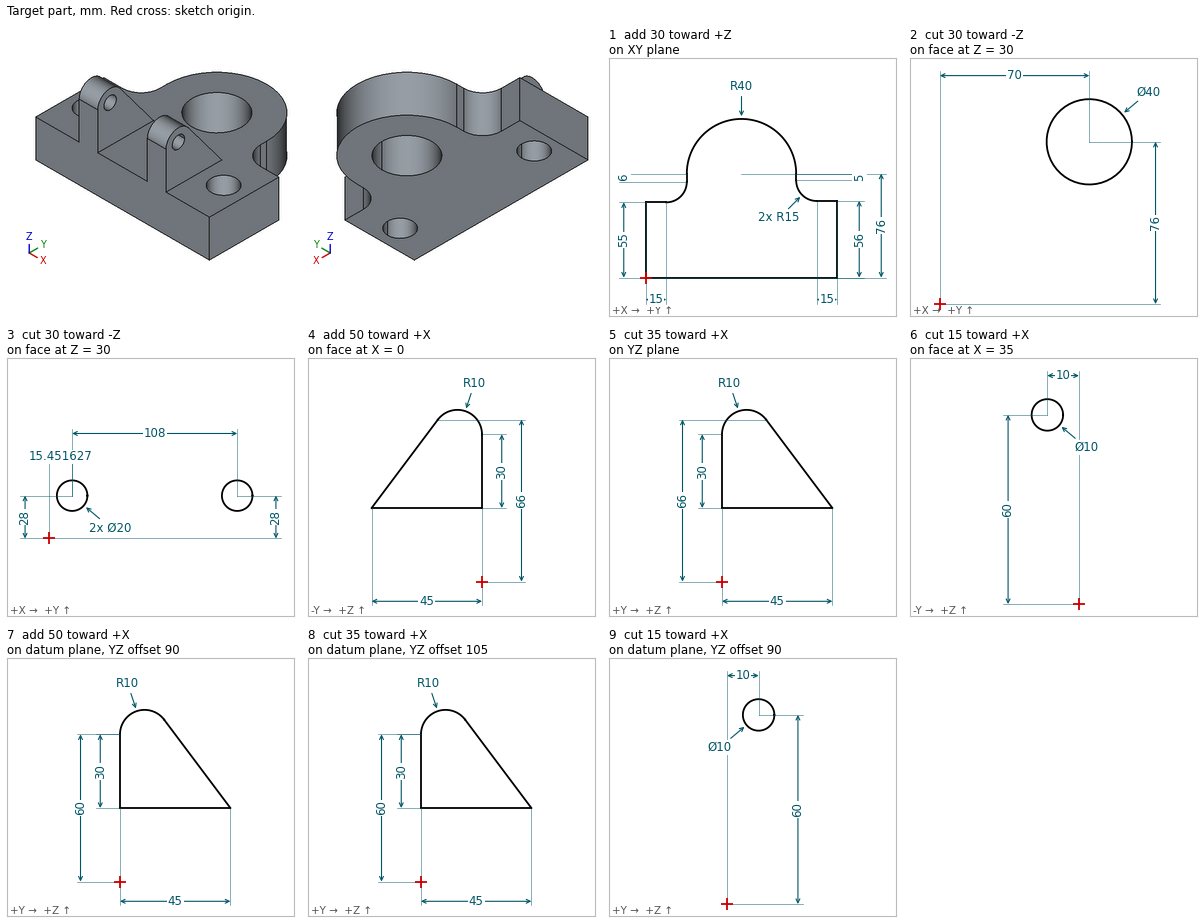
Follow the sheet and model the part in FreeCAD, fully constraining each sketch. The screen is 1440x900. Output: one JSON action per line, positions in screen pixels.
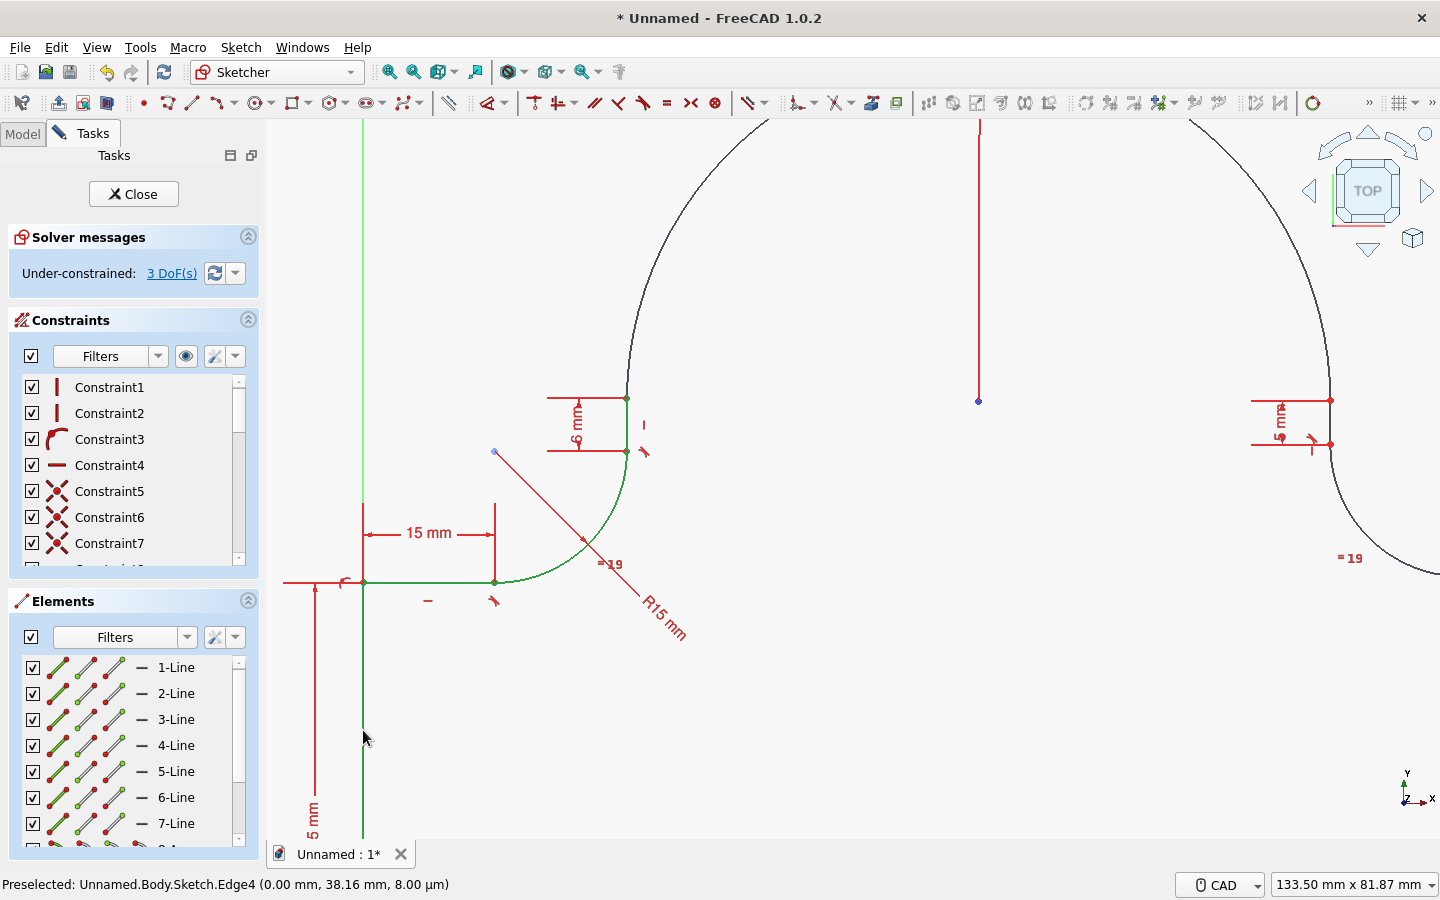
{"action": "scroll", "coordinate": [626, 416], "scroll_direction": "down", "scroll_amount": 4}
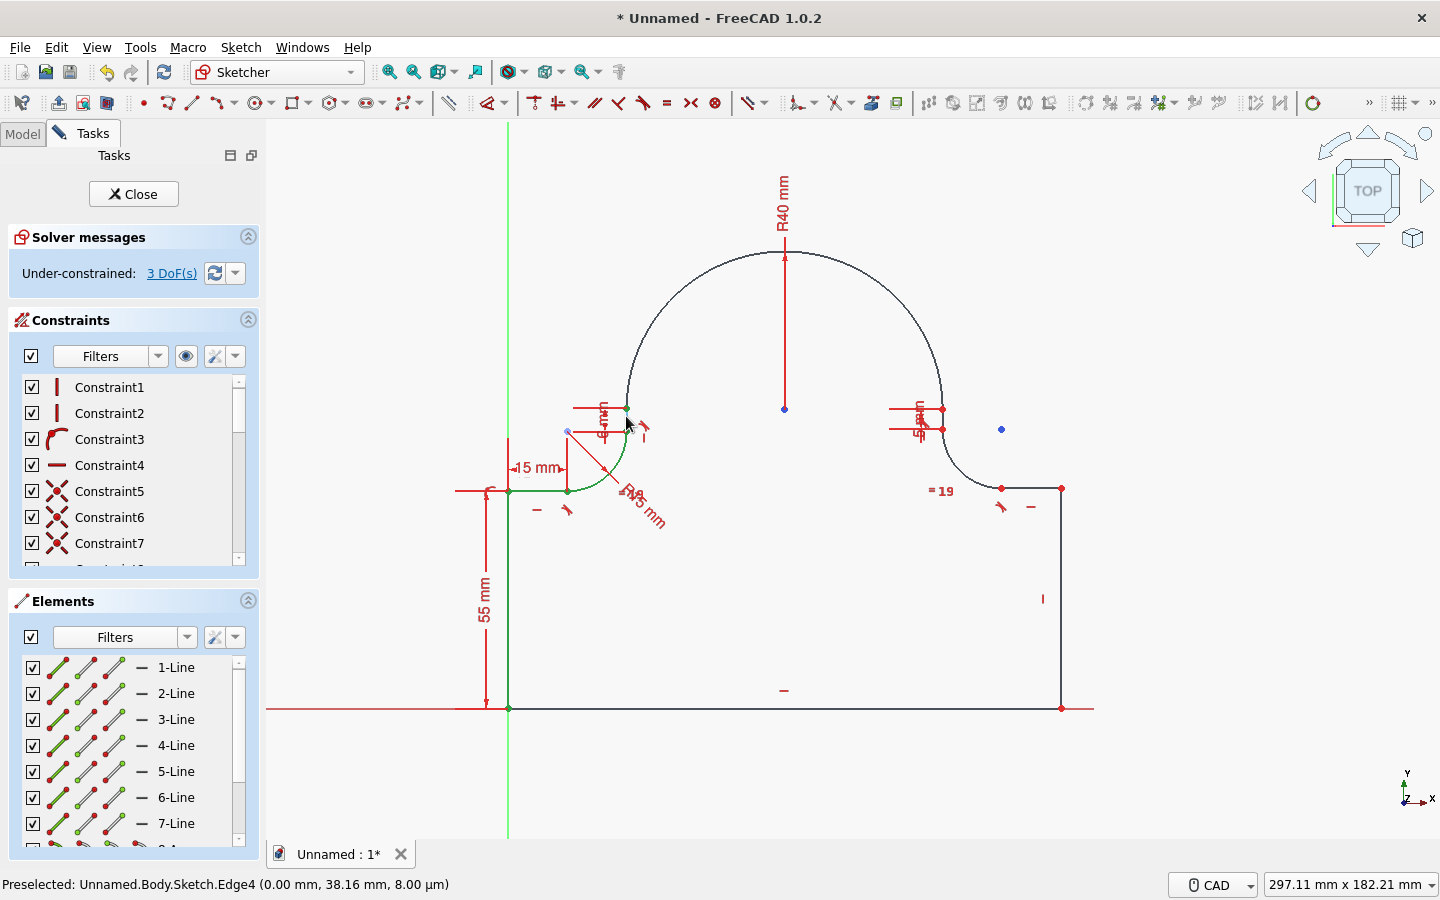
{"action": "left_click", "coordinate": [1061, 642]}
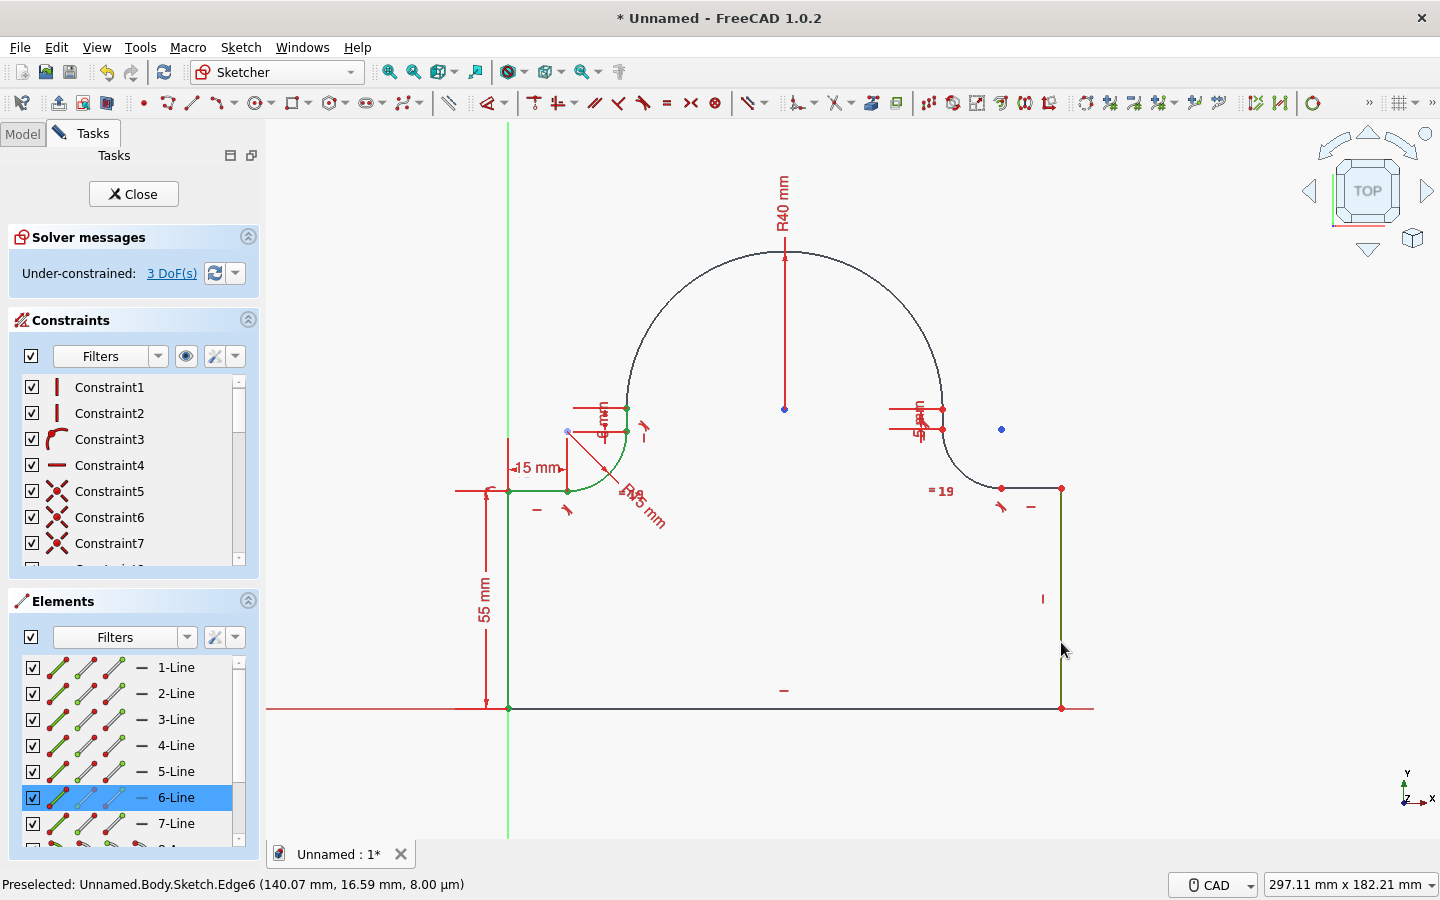
{"action": "left_click", "coordinate": [506, 104]}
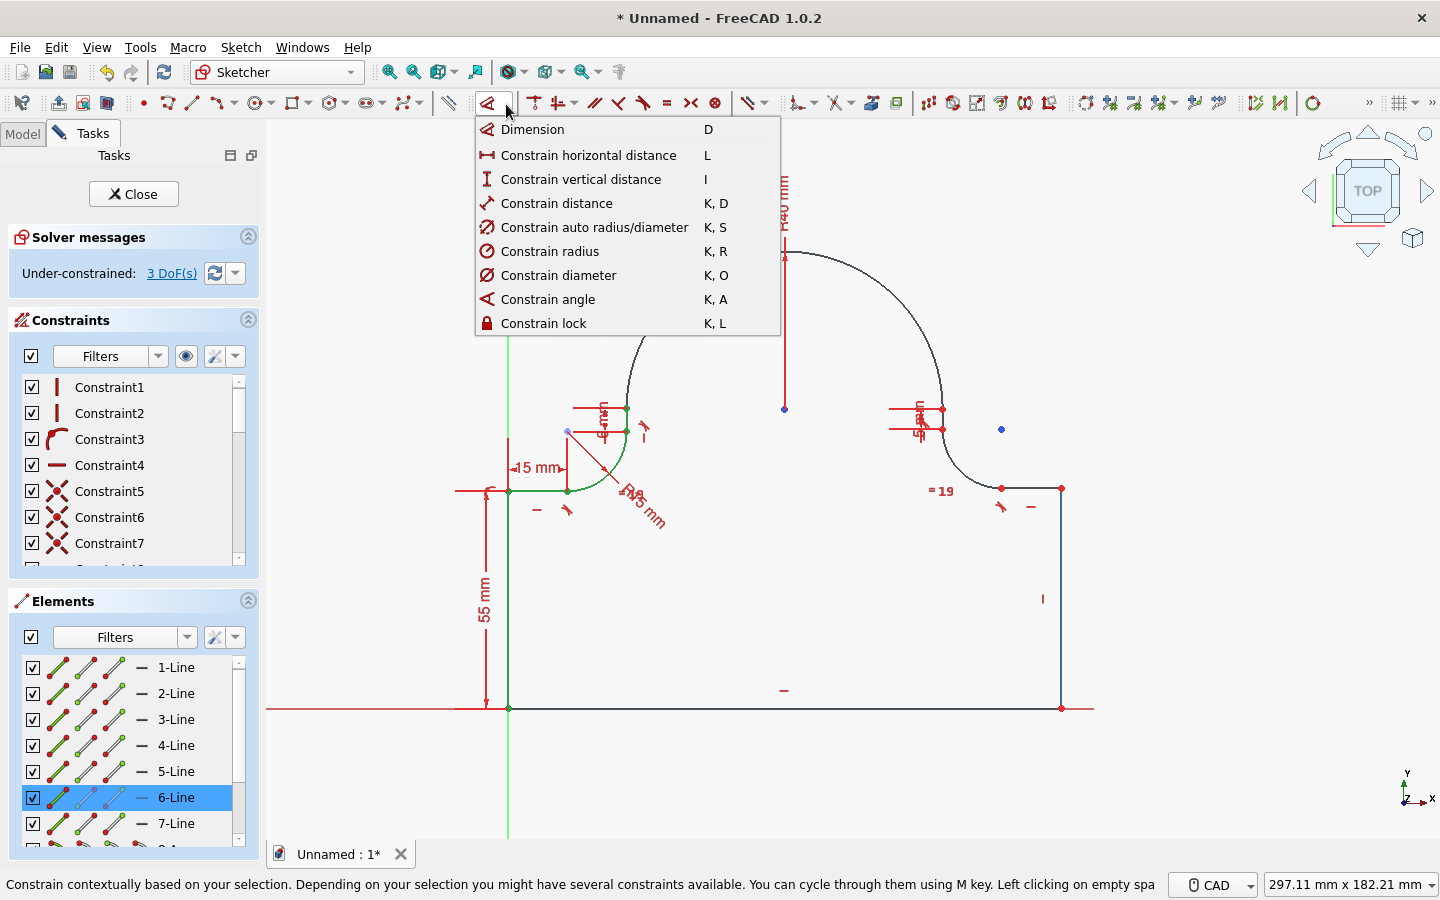
{"action": "left_click", "coordinate": [628, 179]}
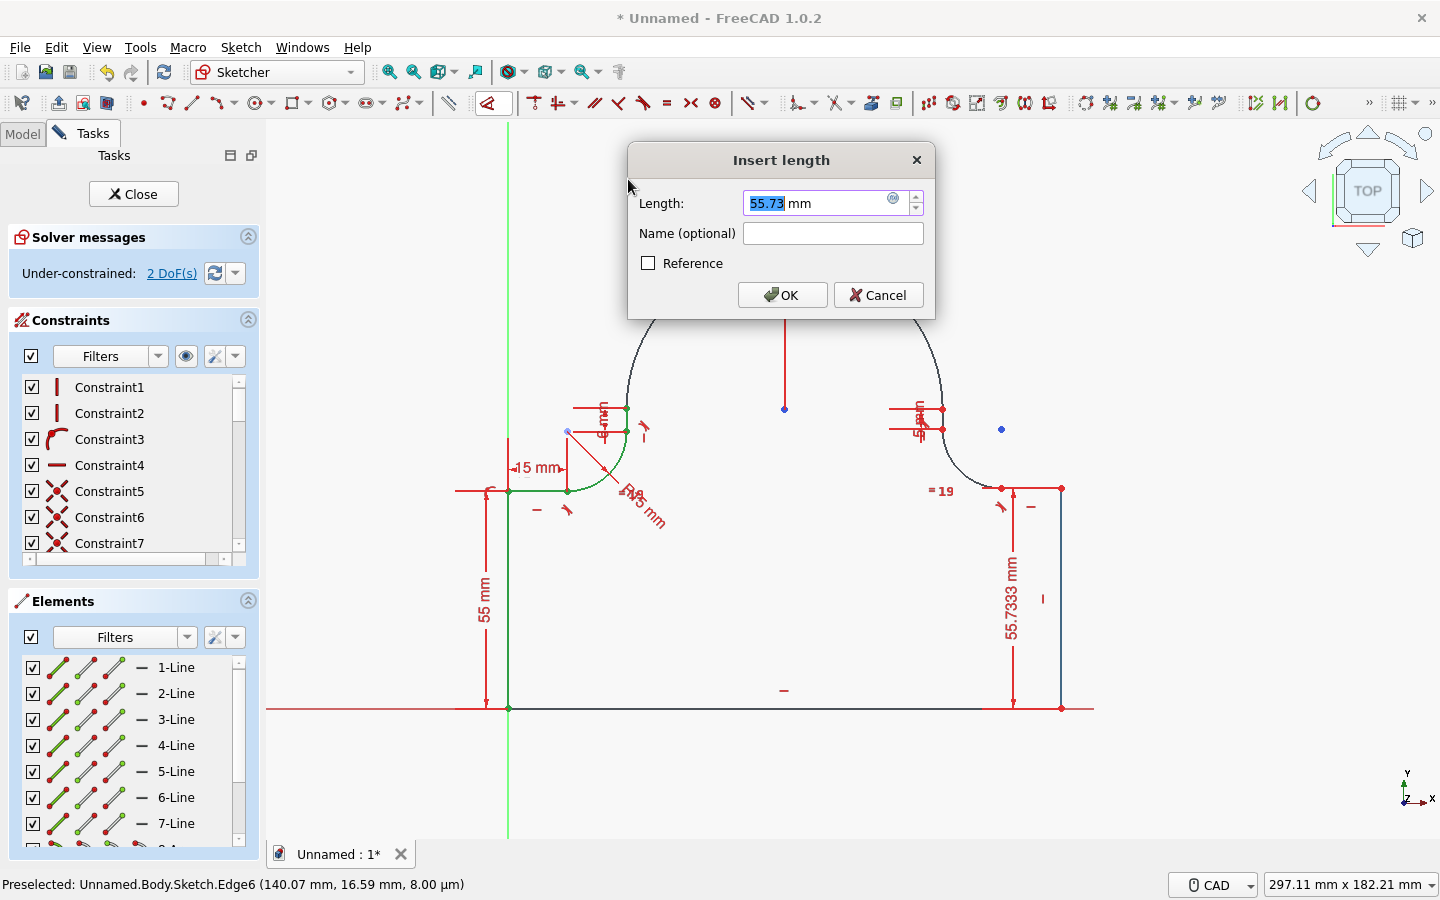
{"action": "type", "text": "56"}
{"action": "key", "text": "Return"}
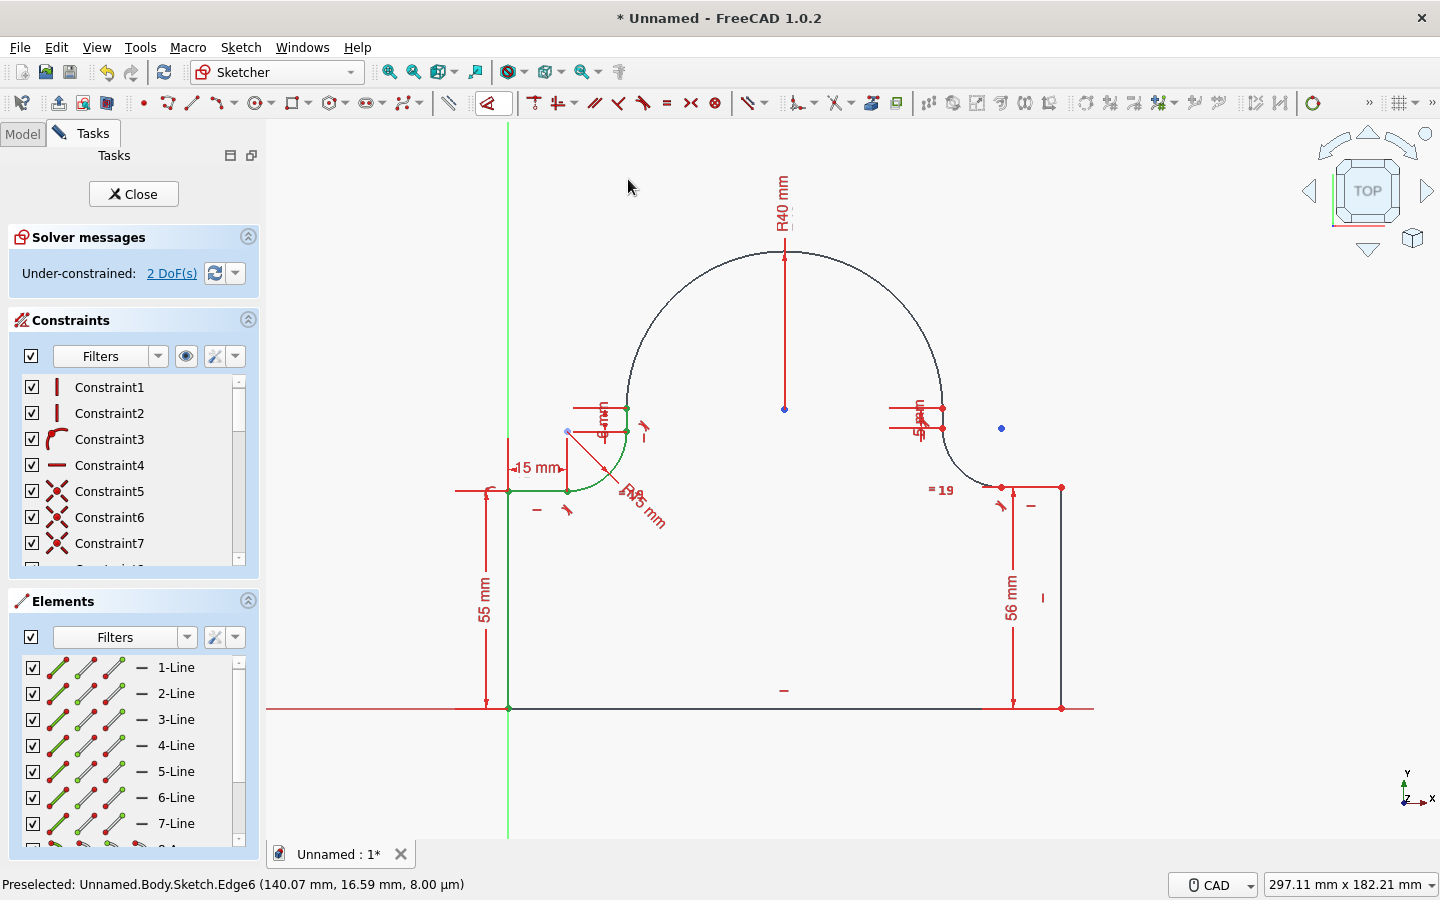
{"action": "left_click", "coordinate": [1044, 487]}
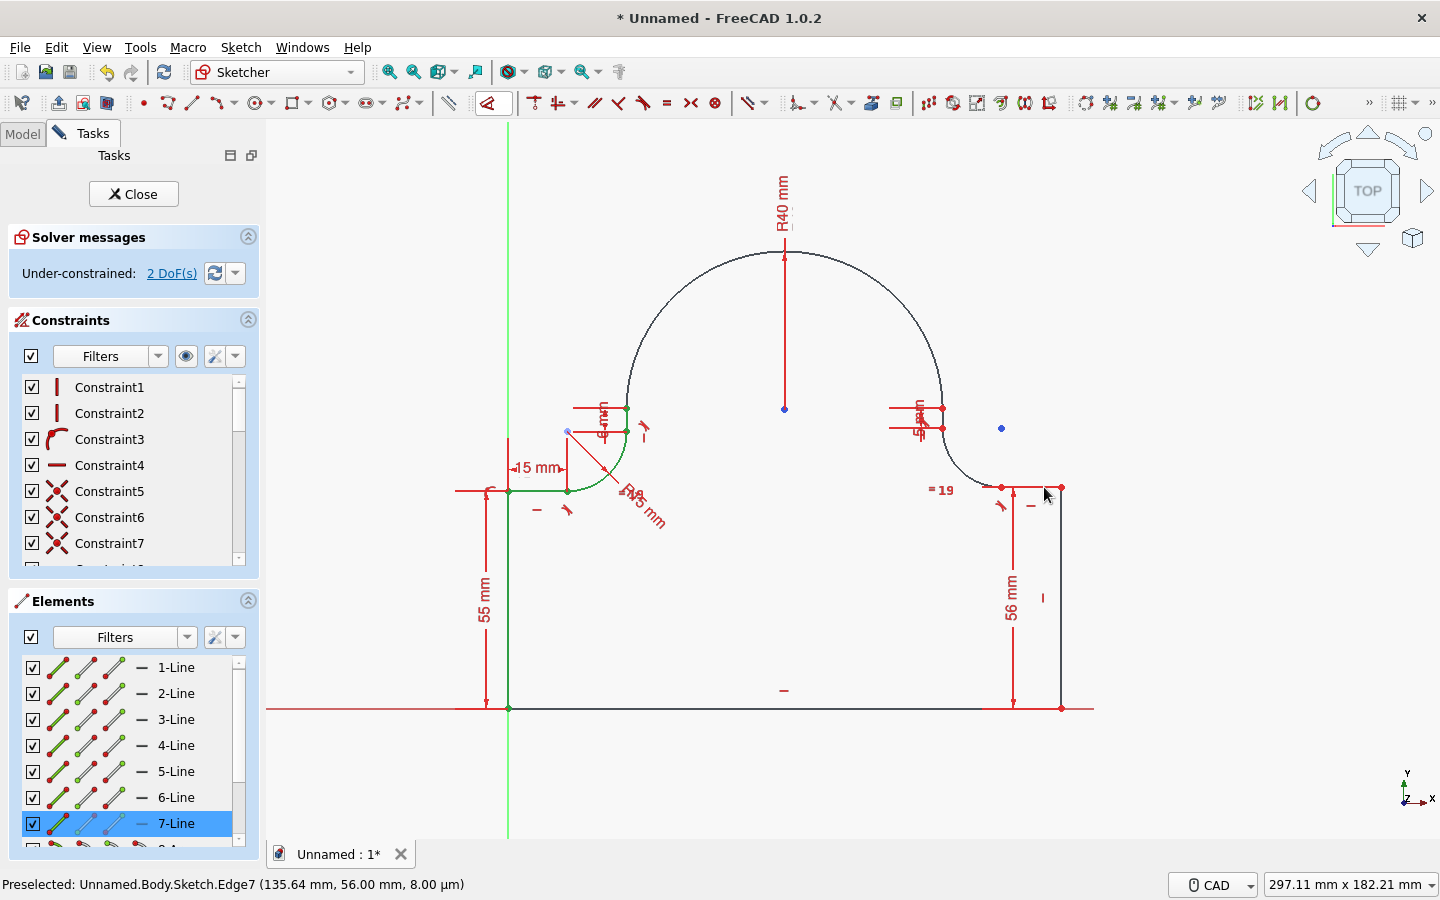
{"action": "key", "text": "l"}